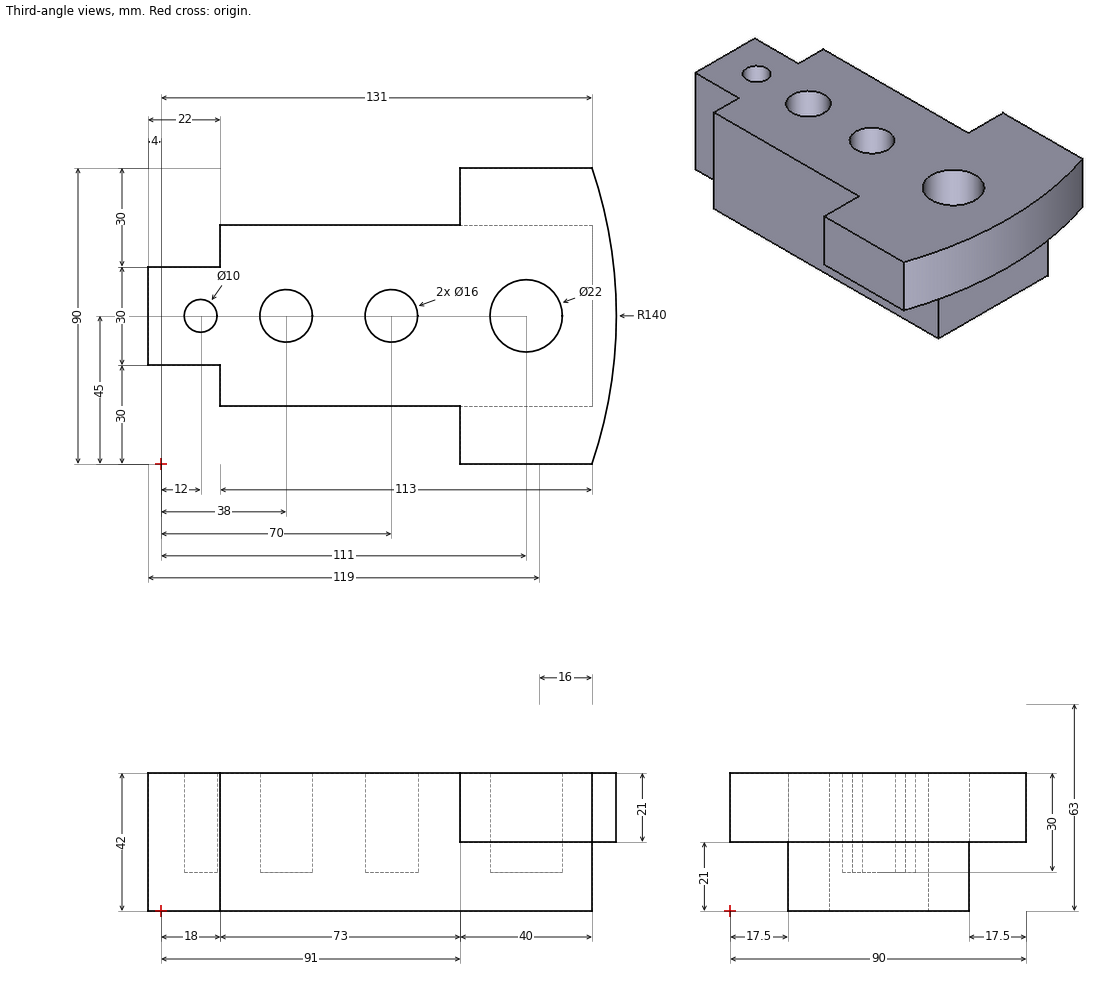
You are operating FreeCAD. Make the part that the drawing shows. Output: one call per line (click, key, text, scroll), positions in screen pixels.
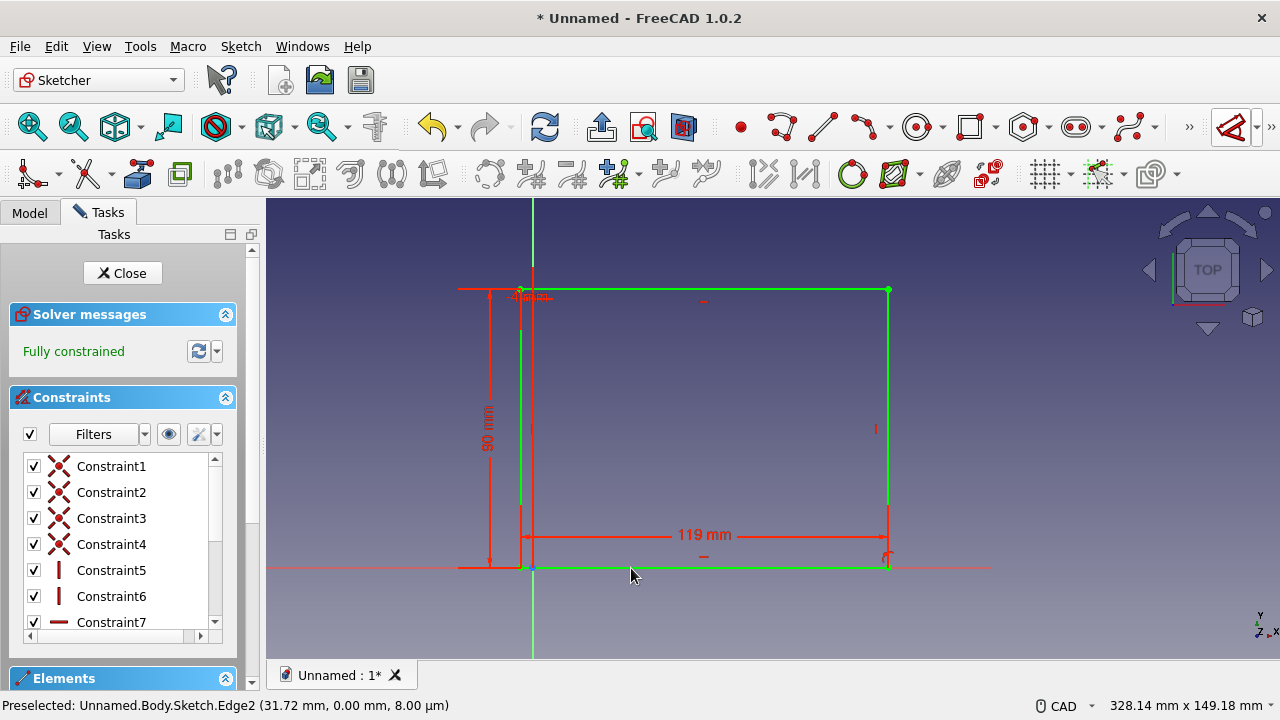
click(123, 273)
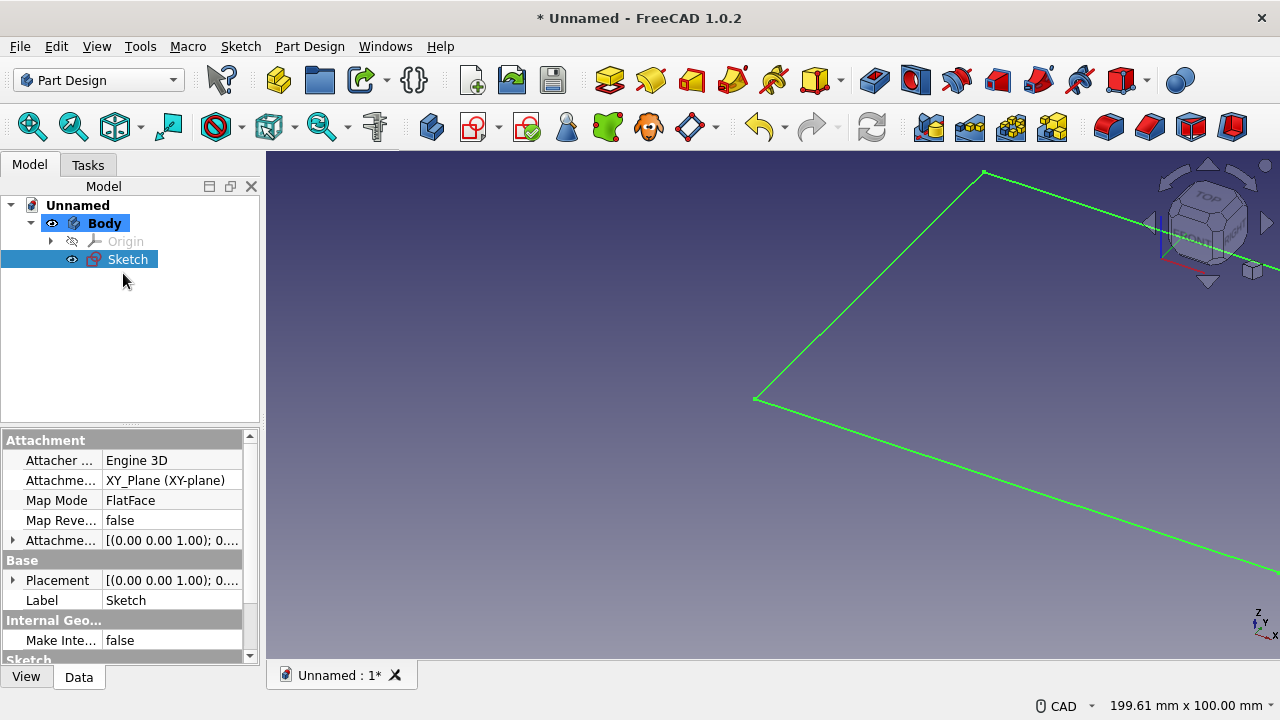
click(610, 80)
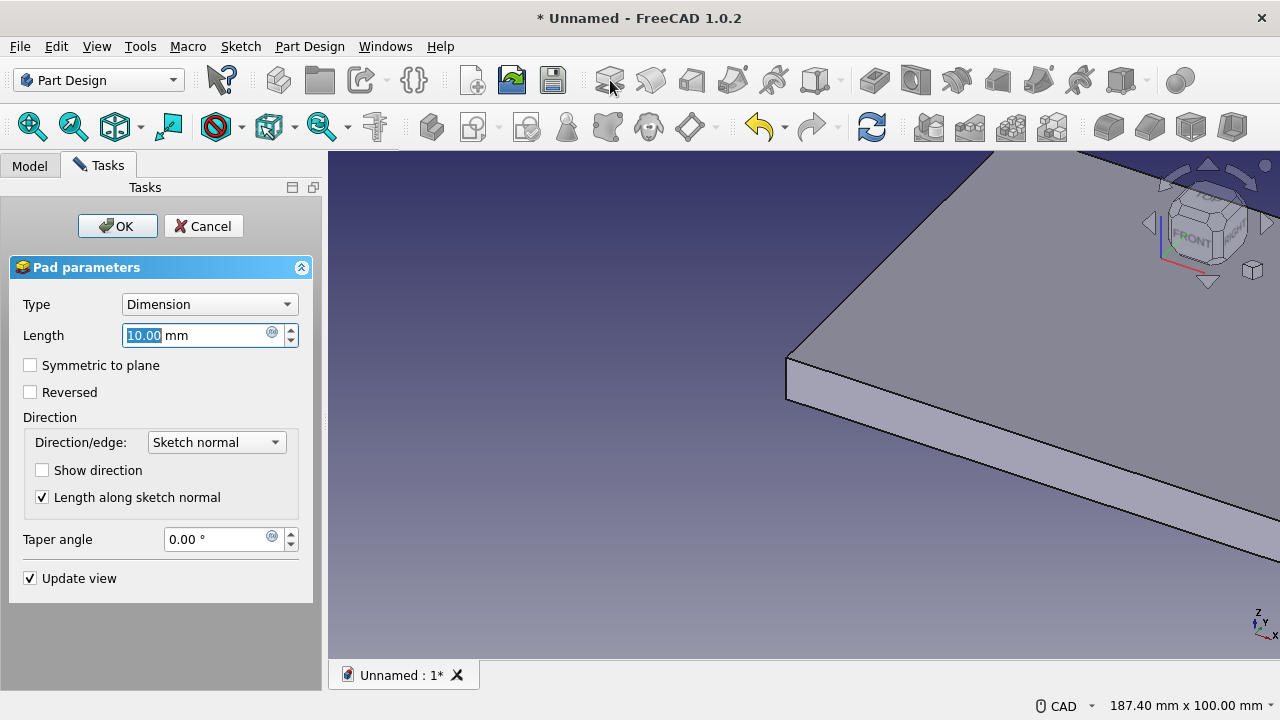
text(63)
key(Tab)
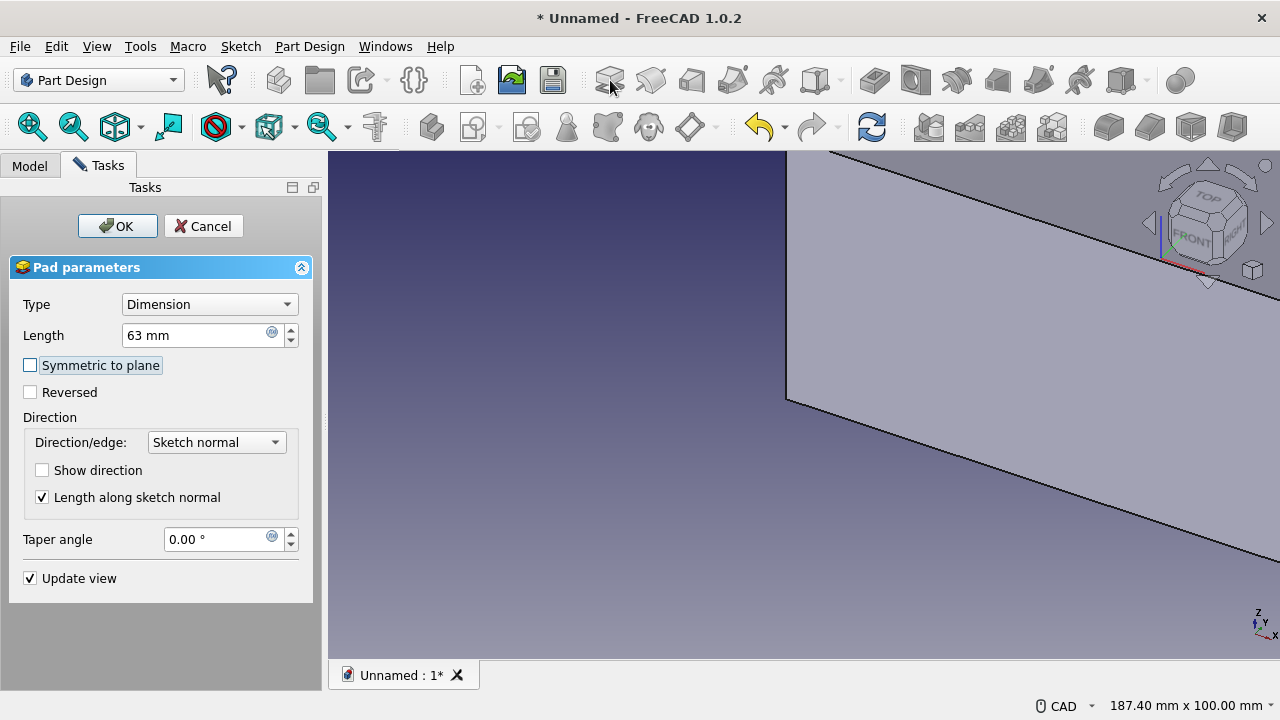
click(118, 226)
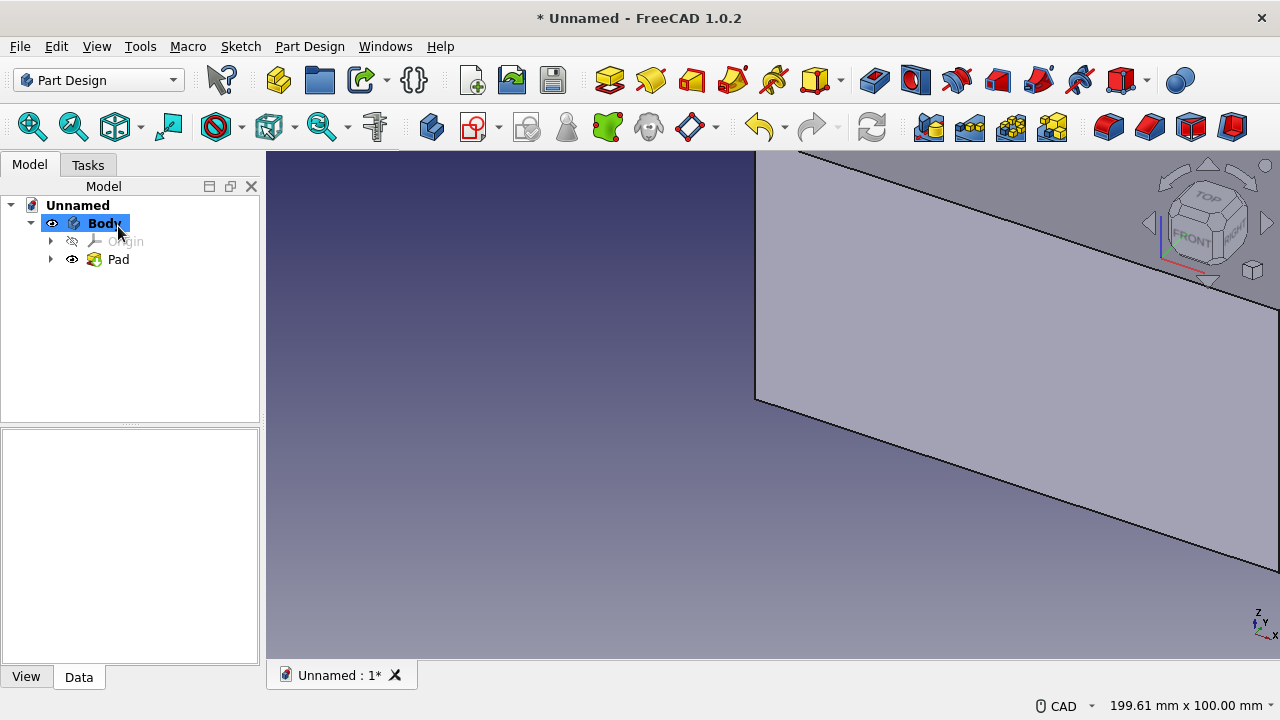
click(33, 128)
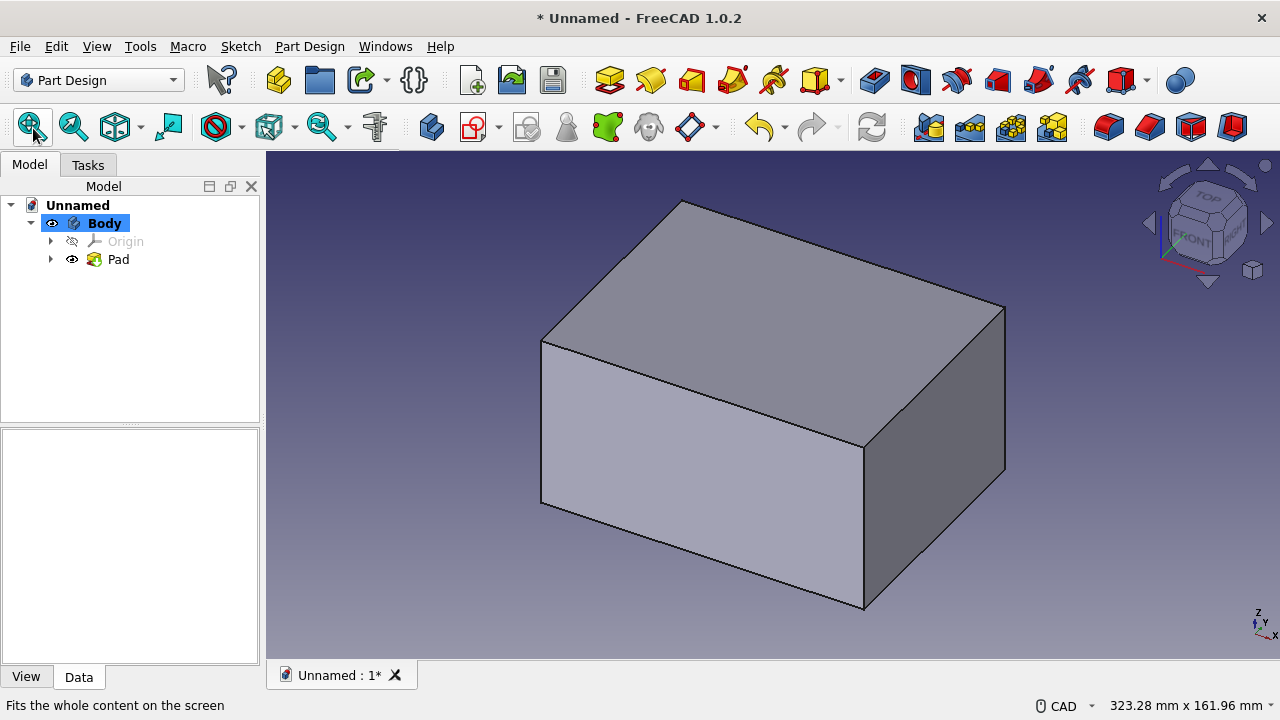
click(773, 323)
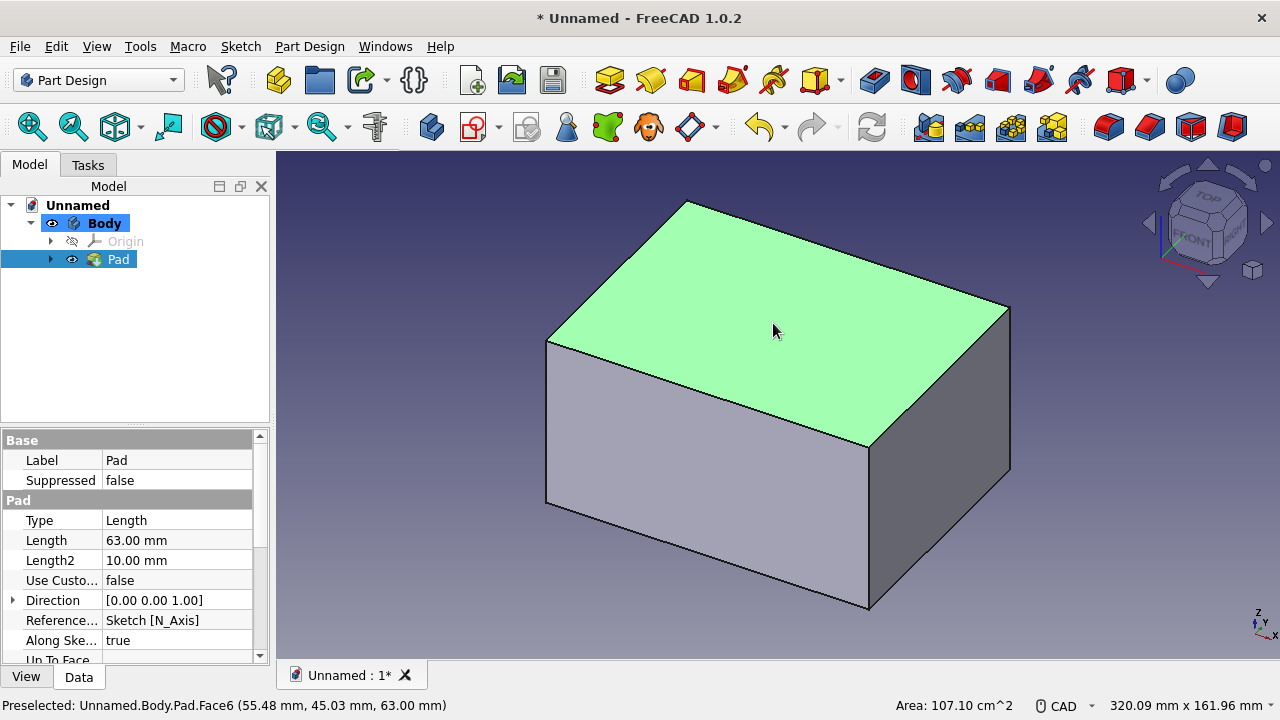
click(472, 128)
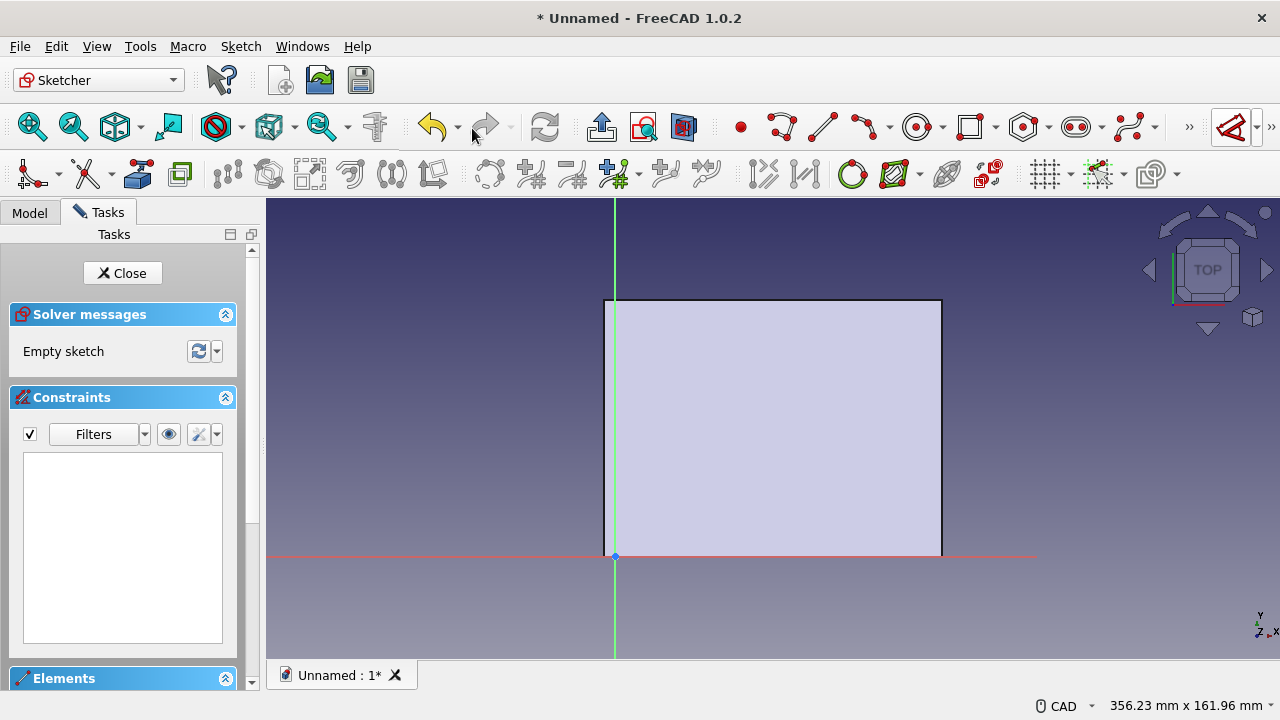
click(970, 128)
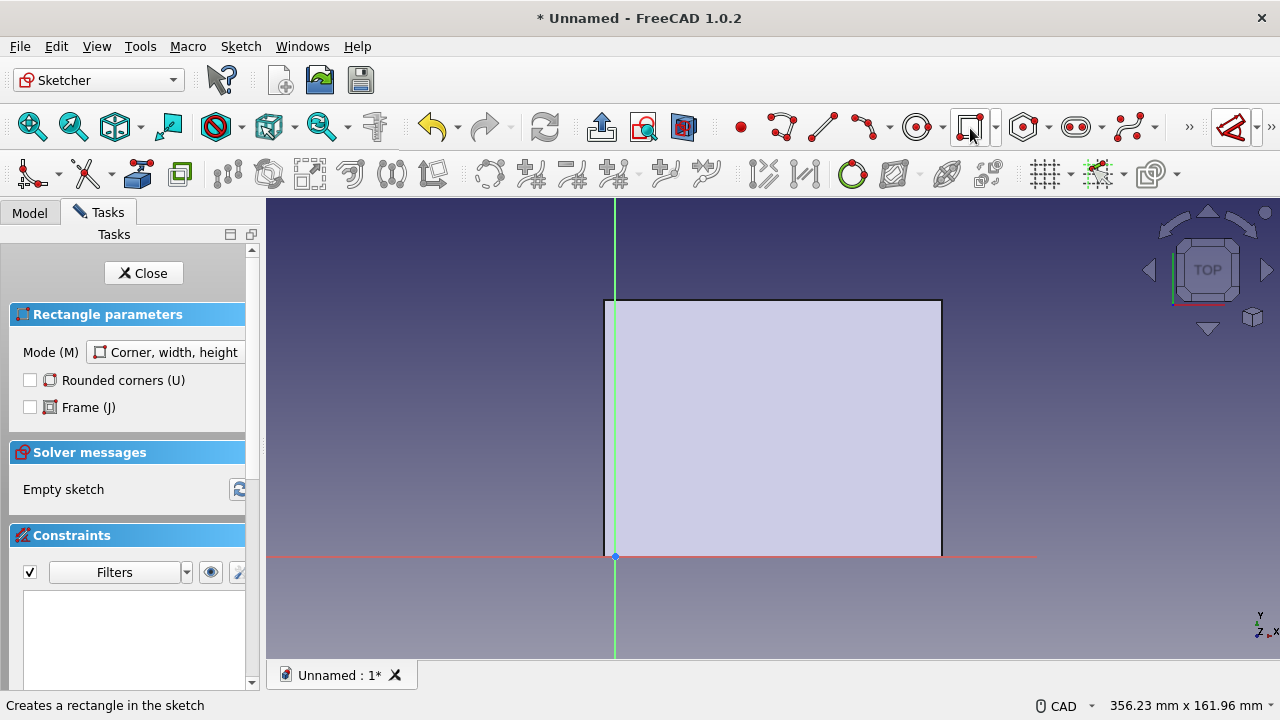
scroll(604, 300, up, 2)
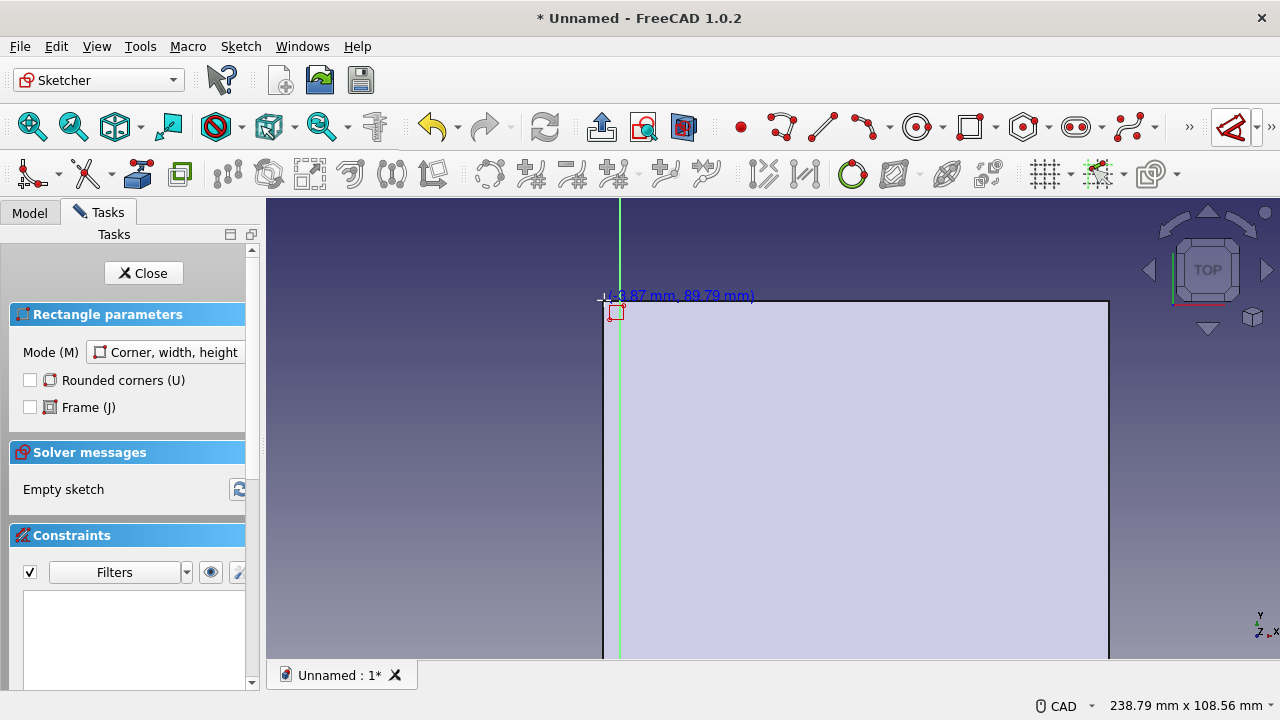
click(603, 301)
move(697, 428)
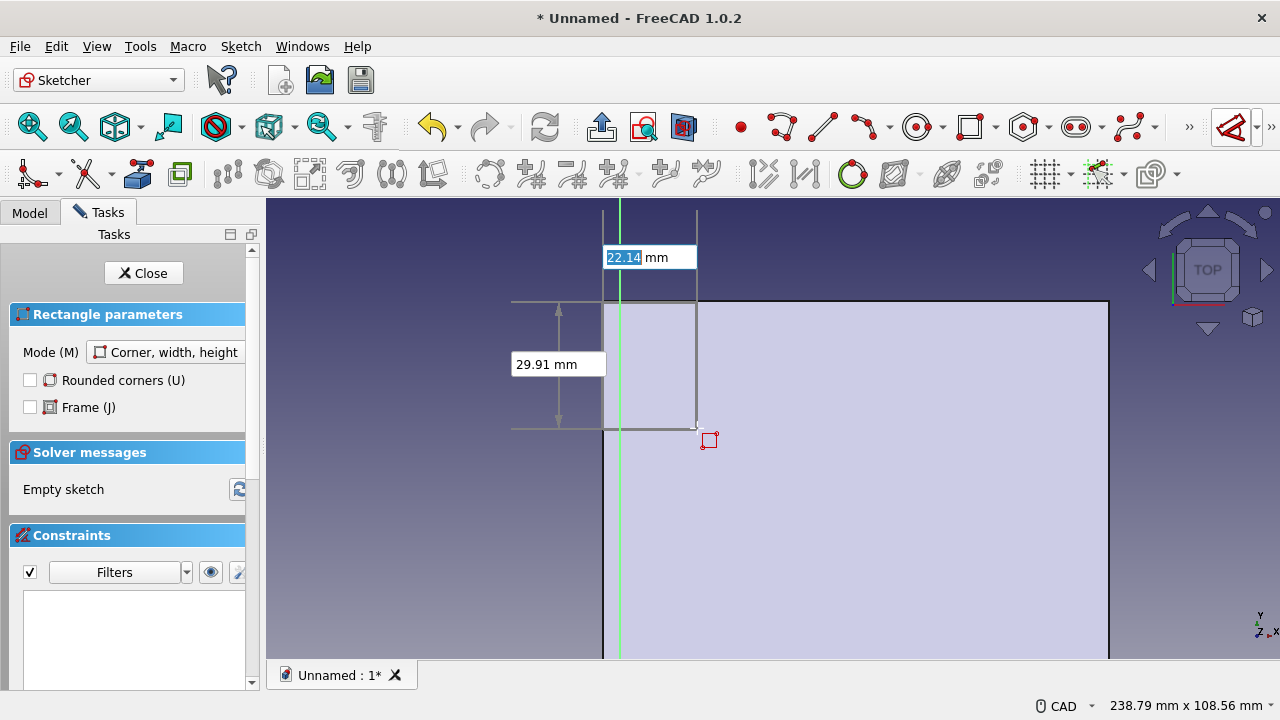
text(22)
key(Tab)
text(30)
key(Return)